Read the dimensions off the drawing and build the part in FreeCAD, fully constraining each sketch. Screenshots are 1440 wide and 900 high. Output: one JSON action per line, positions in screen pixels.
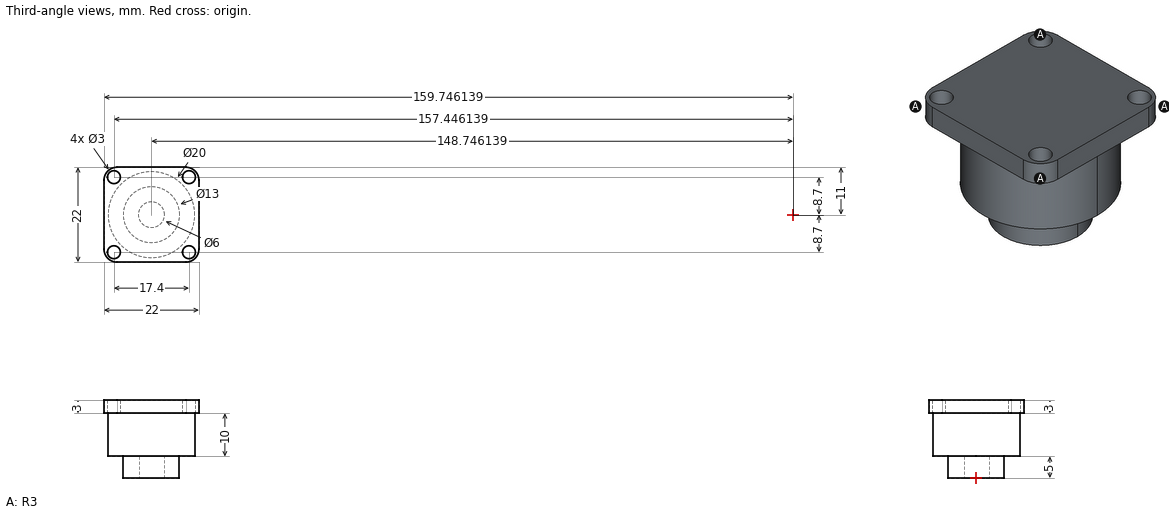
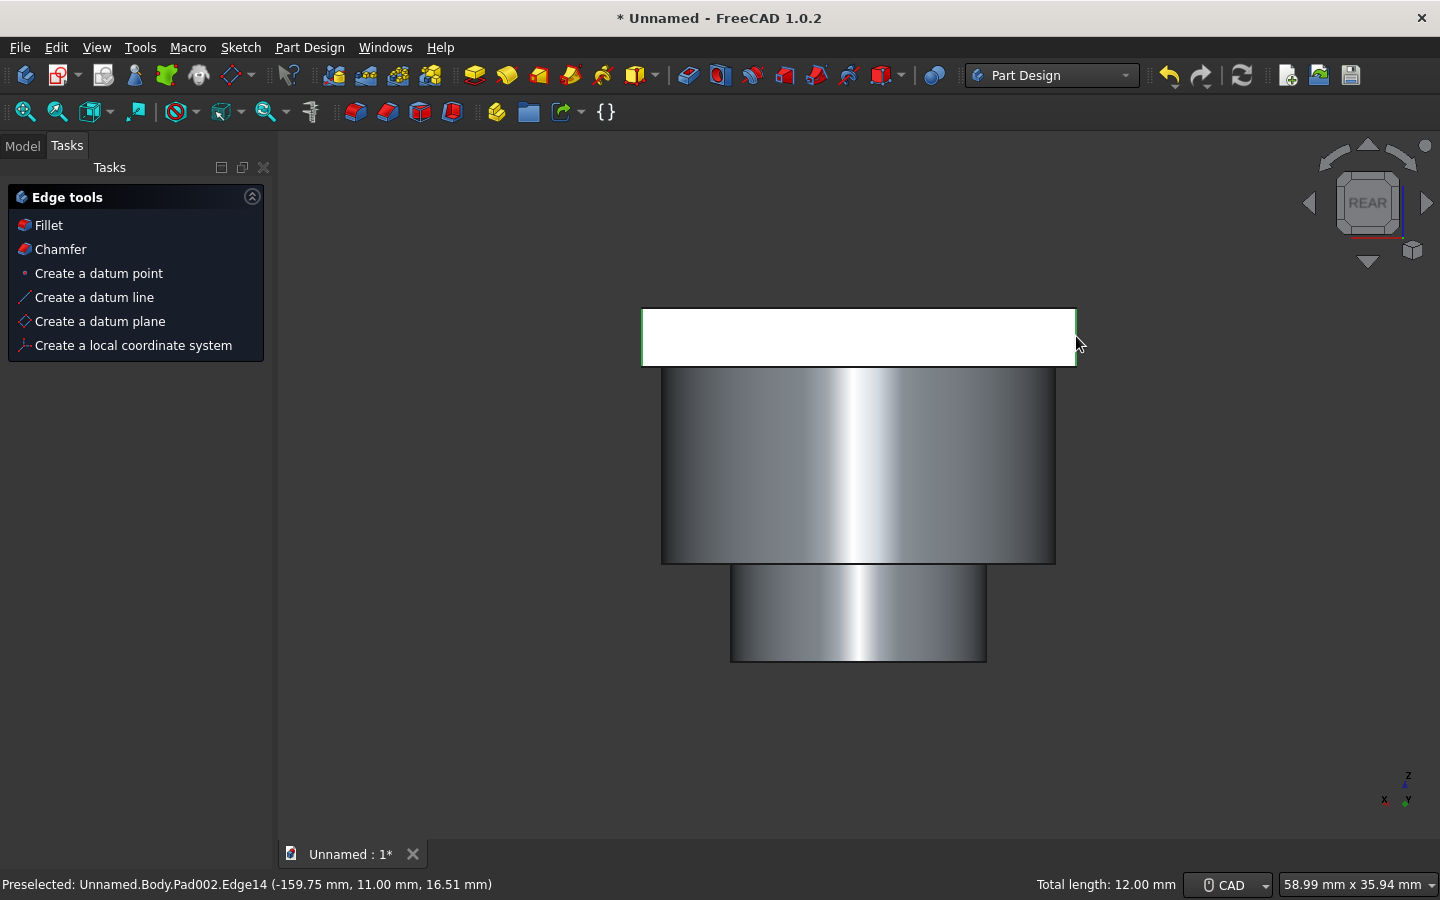
{"action": "left_click", "coordinate": [356, 112]}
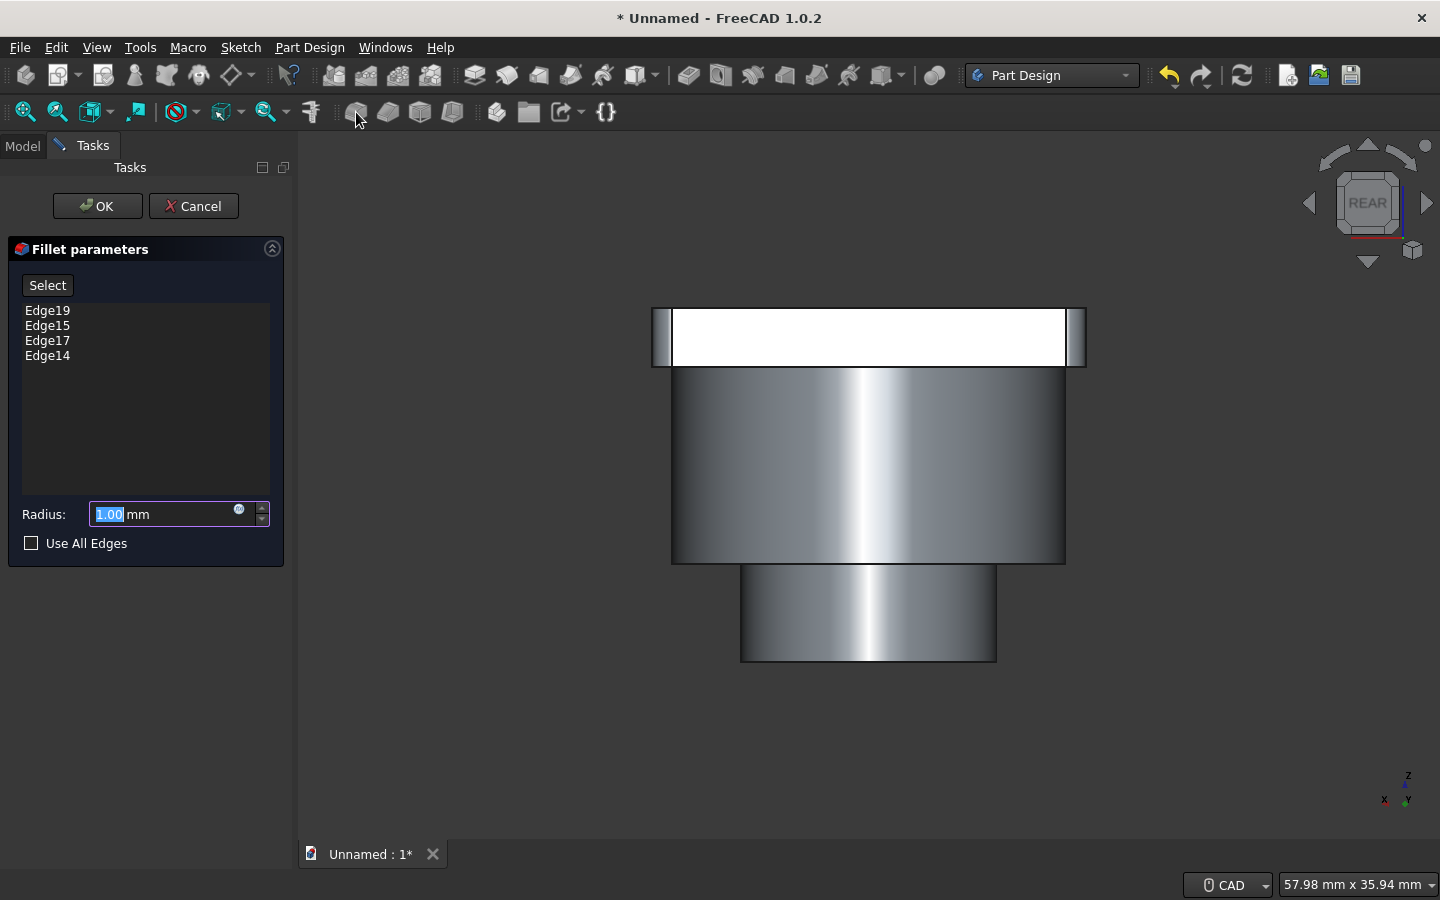
{"action": "type", "text": "3"}
{"action": "key", "text": "Tab"}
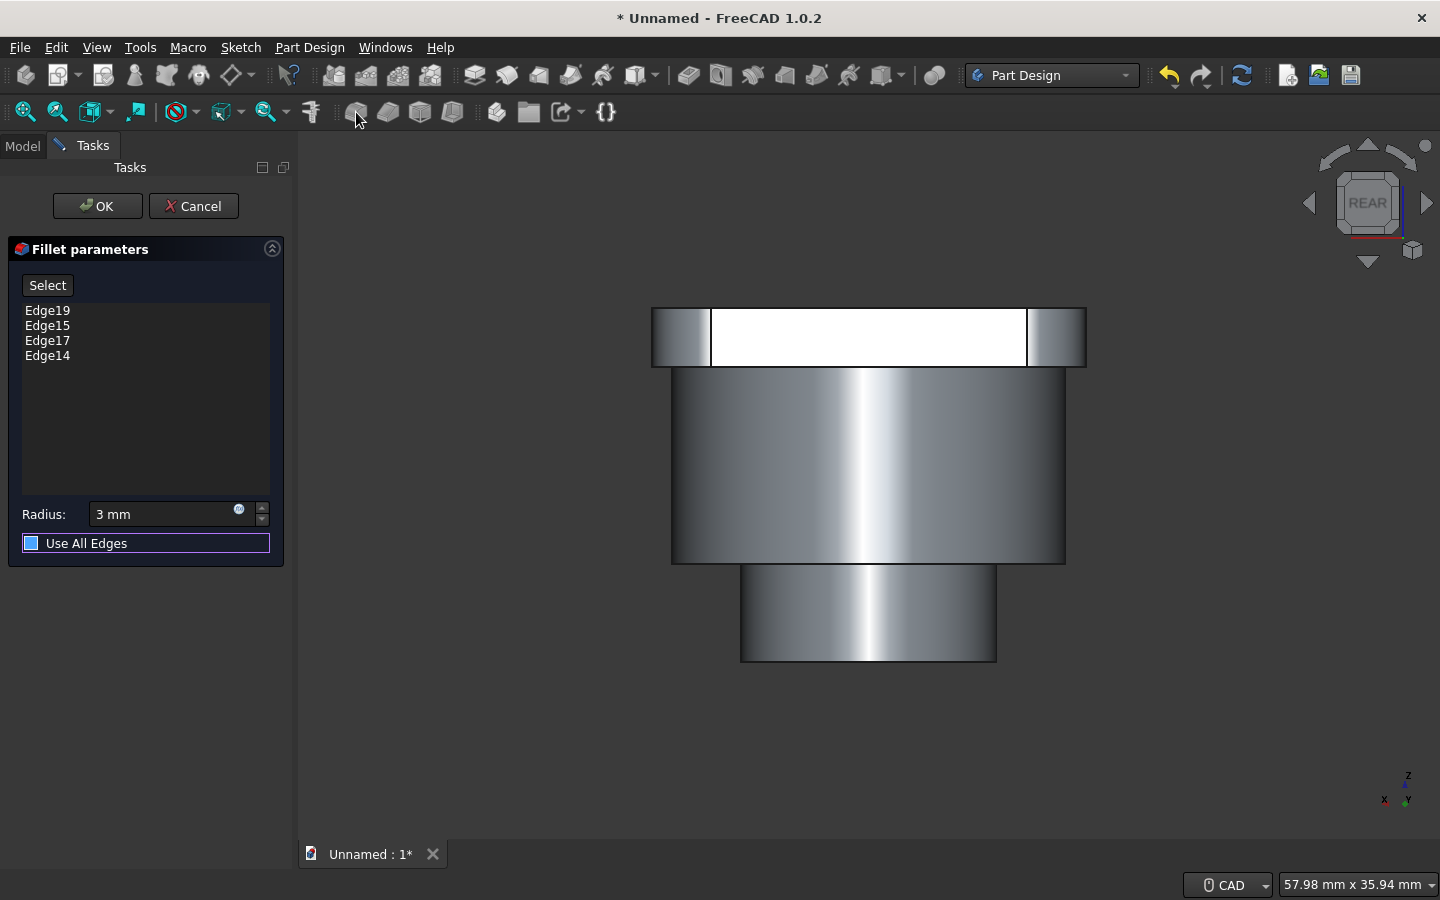
{"action": "left_click", "coordinate": [98, 206]}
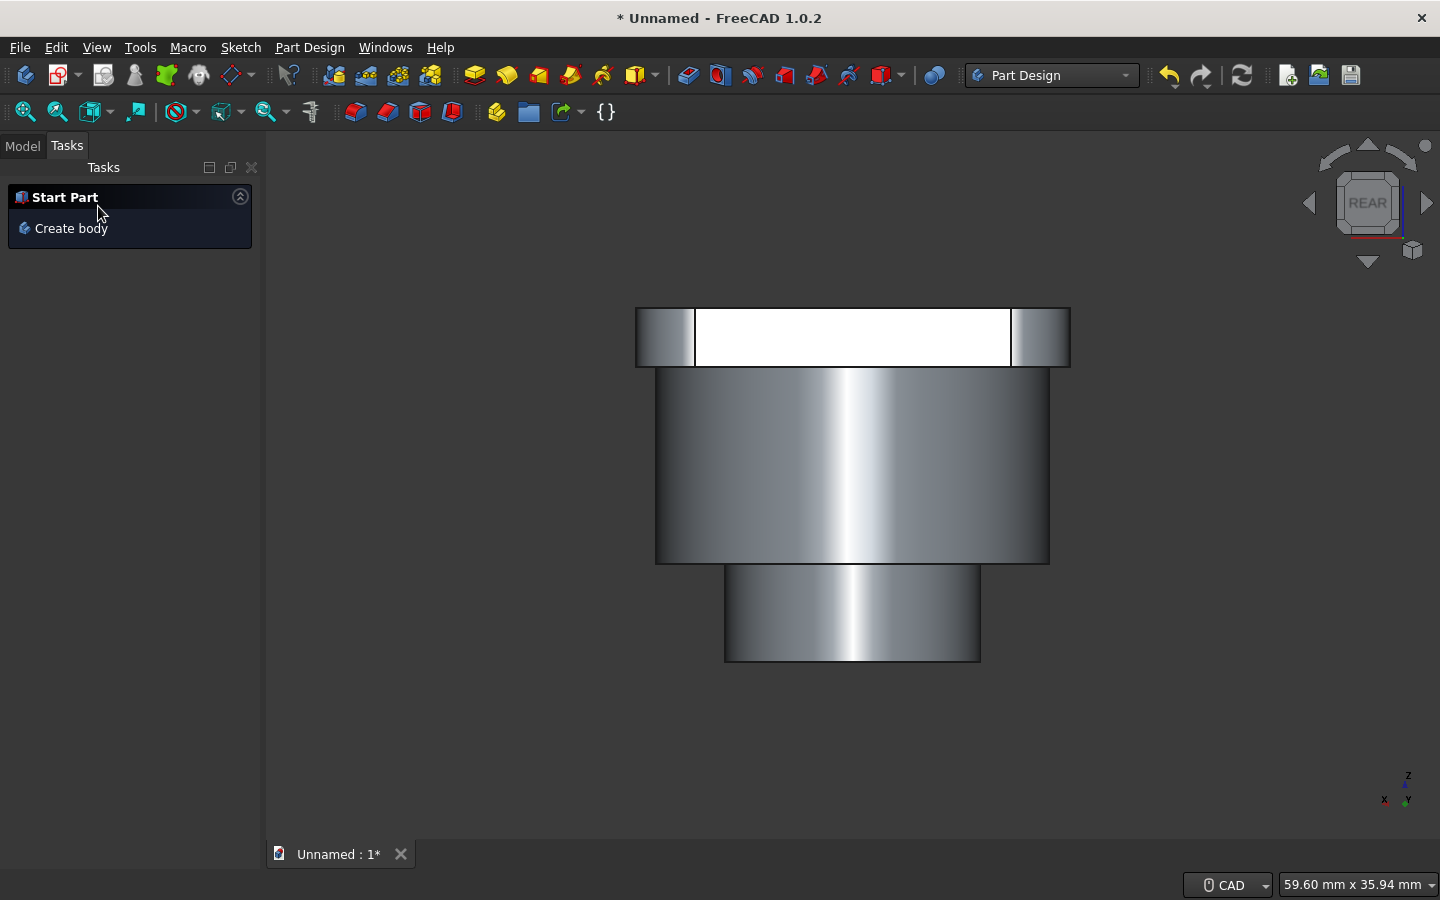
{"action": "key", "text": "5"}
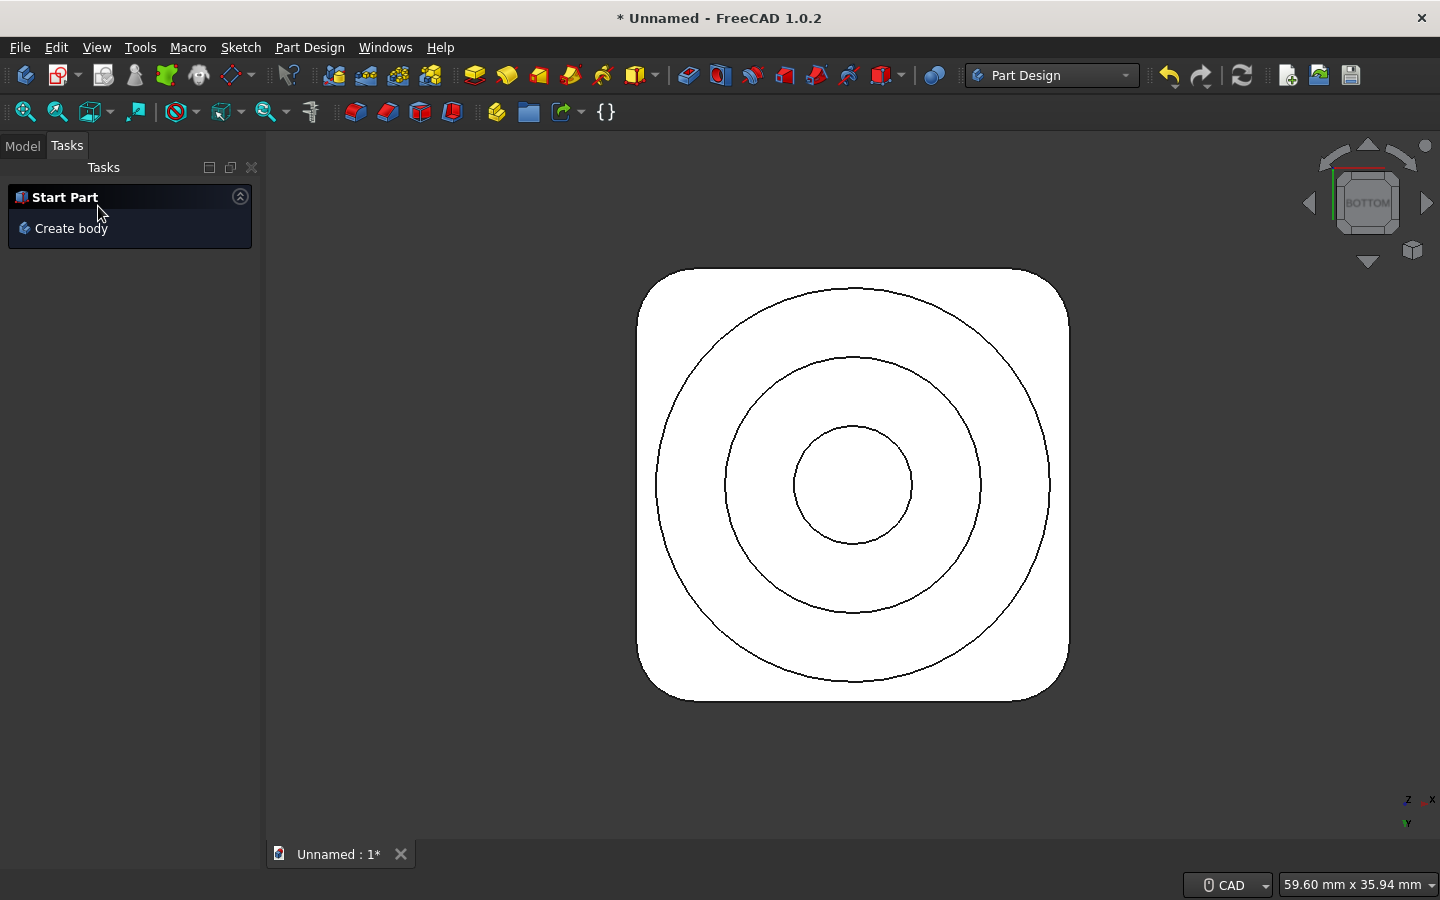
{"action": "left_click", "coordinate": [729, 298]}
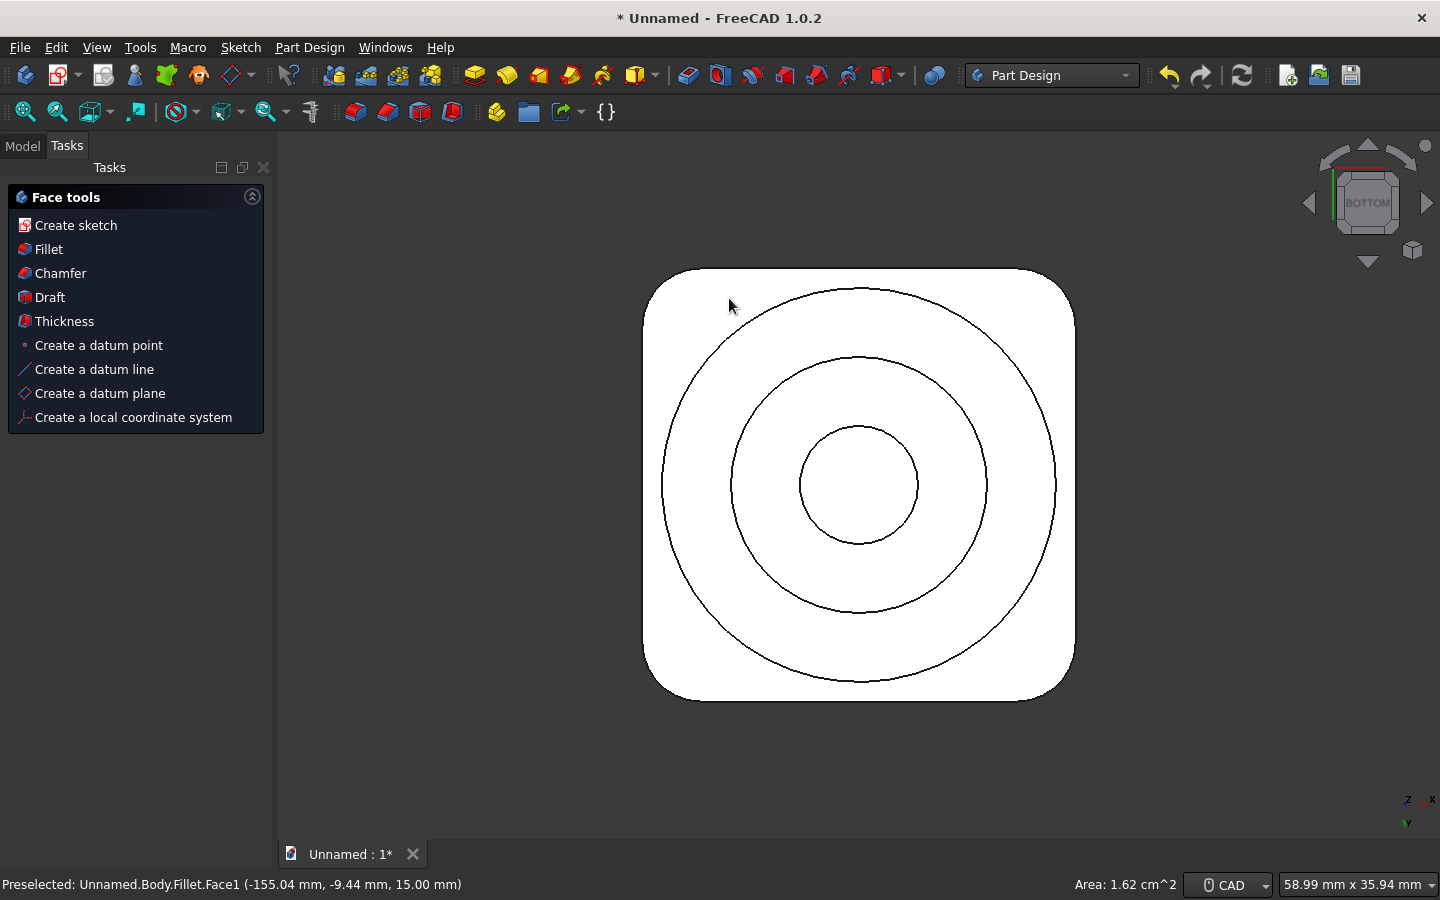
{"action": "left_click", "coordinate": [58, 76]}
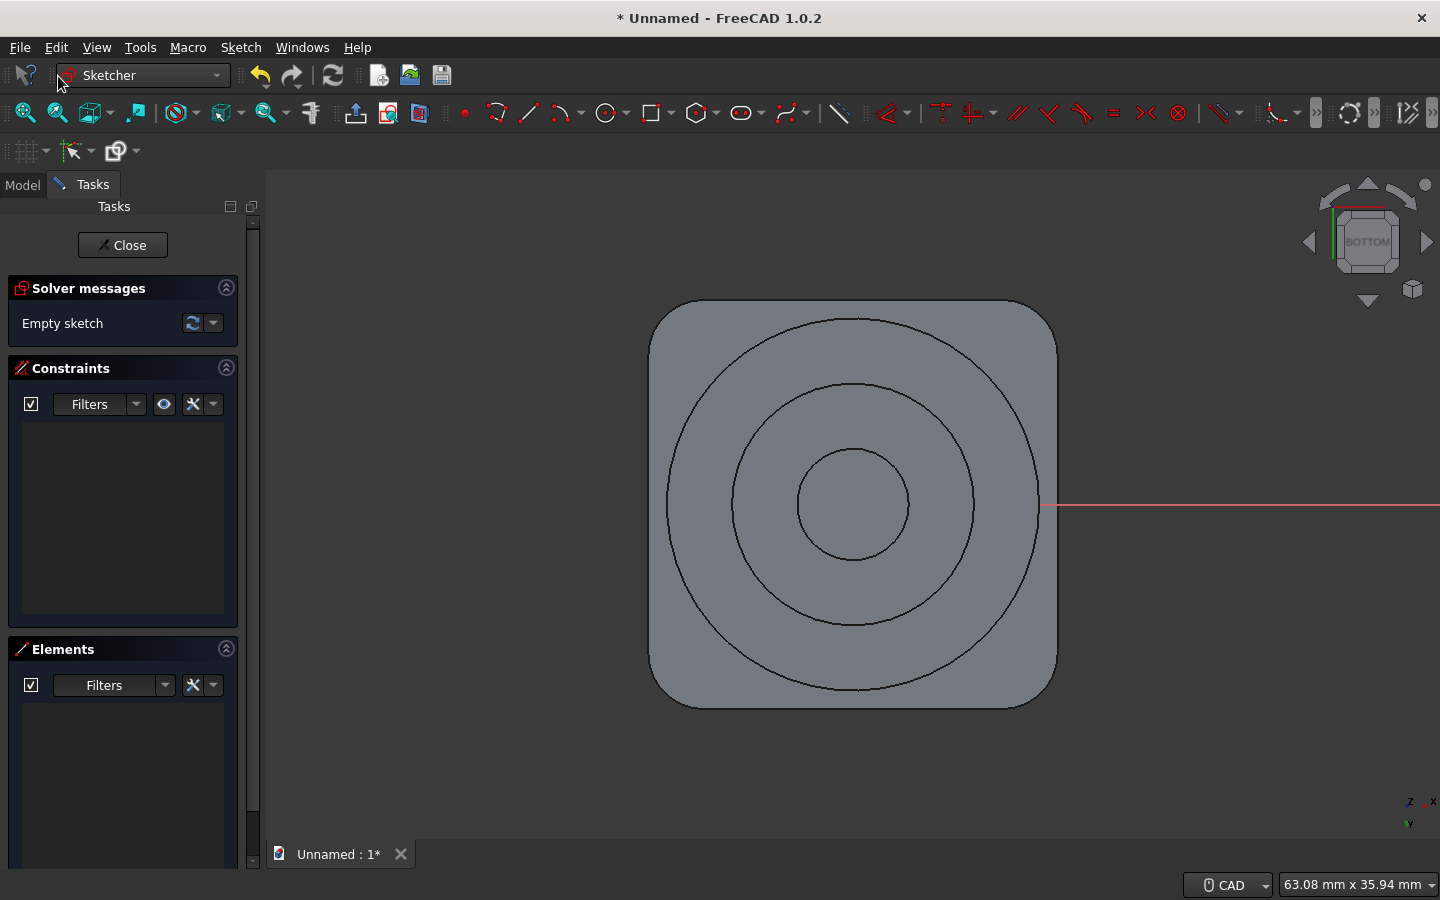
{"action": "left_click", "coordinate": [606, 114]}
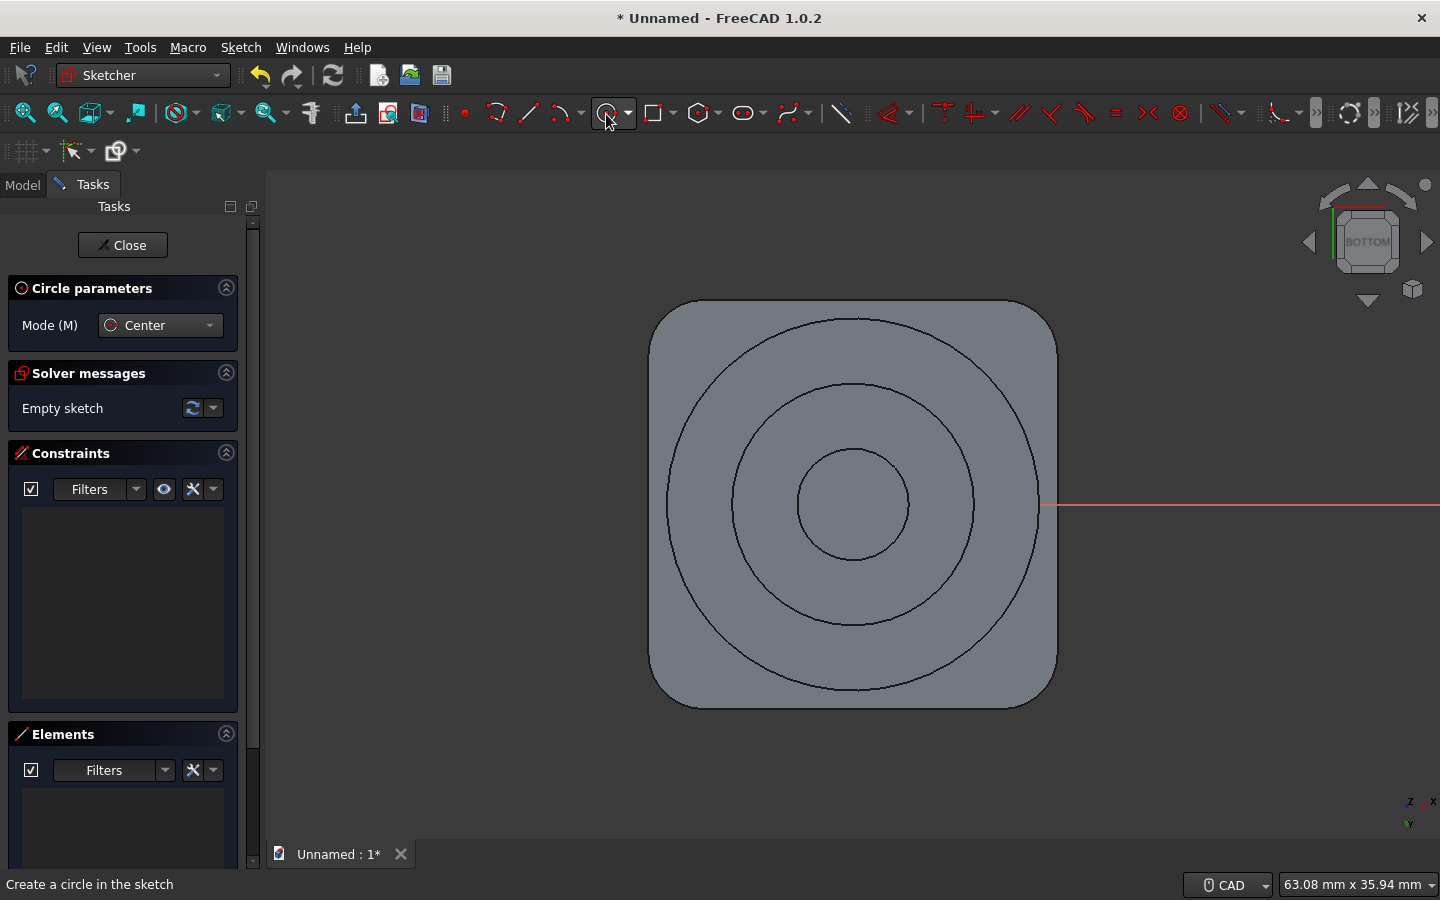
{"action": "left_click", "coordinate": [691, 666]}
{"action": "mouse_move", "coordinate": [711, 647]}